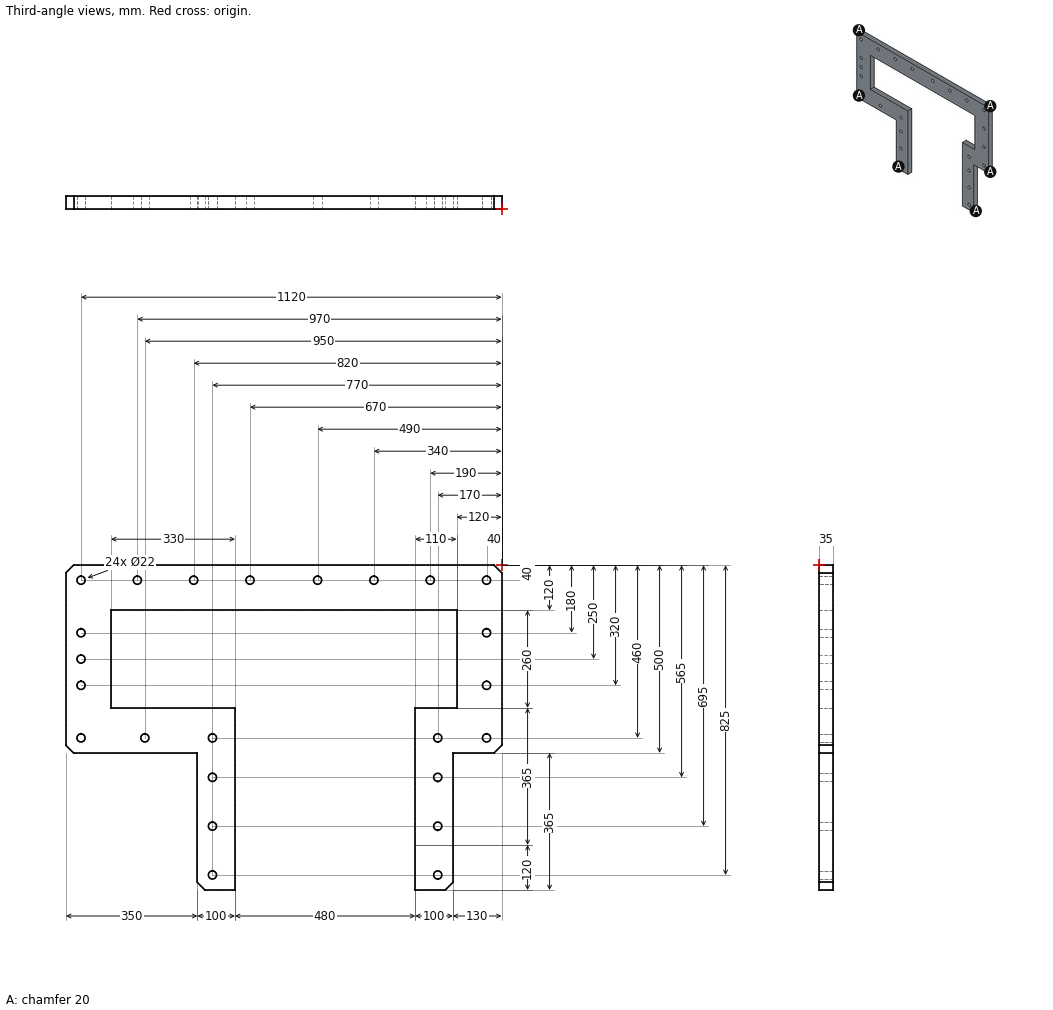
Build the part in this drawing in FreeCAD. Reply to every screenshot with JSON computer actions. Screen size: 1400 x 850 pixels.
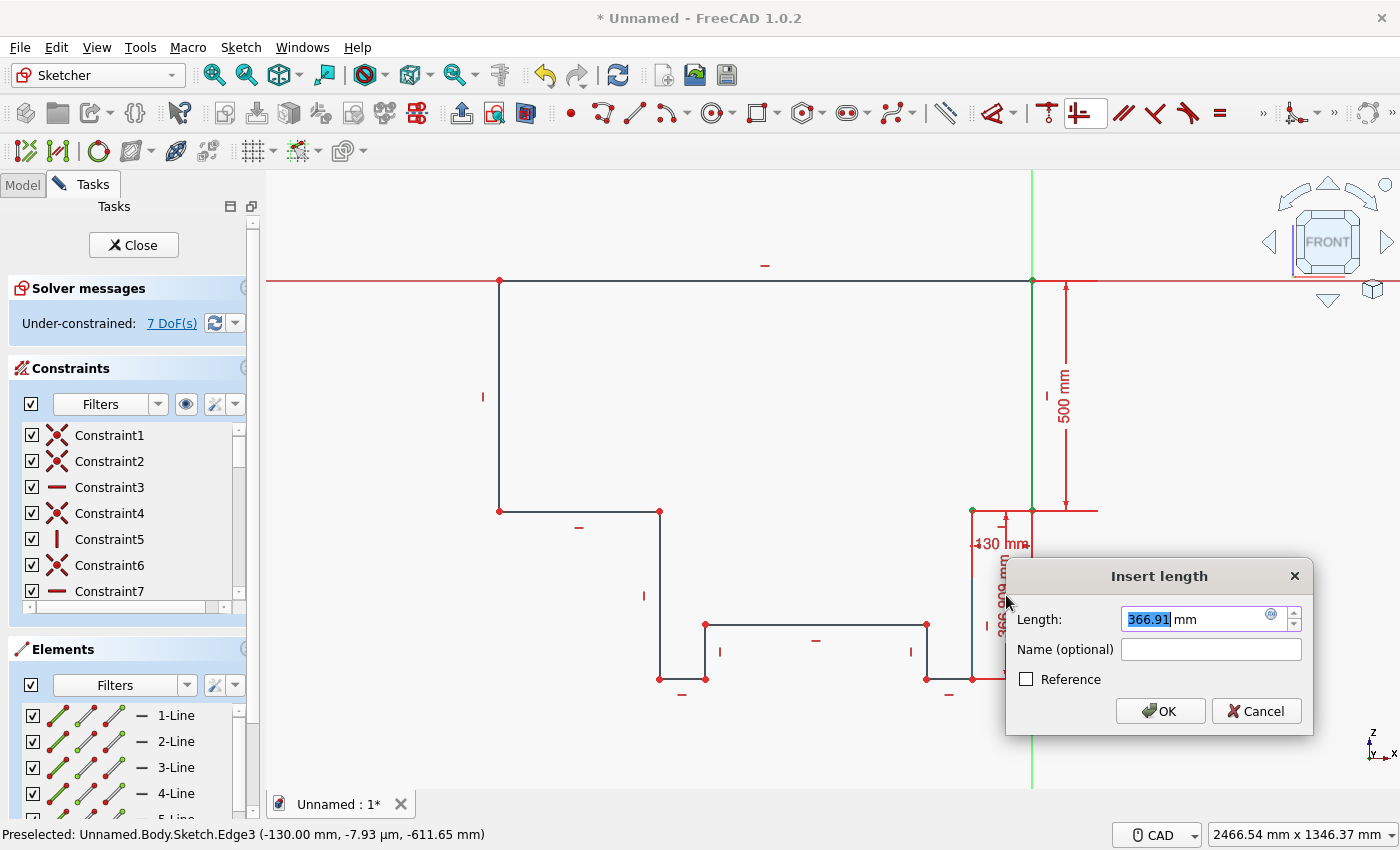
{"action": "type", "text": "365"}
{"action": "key", "text": "Return"}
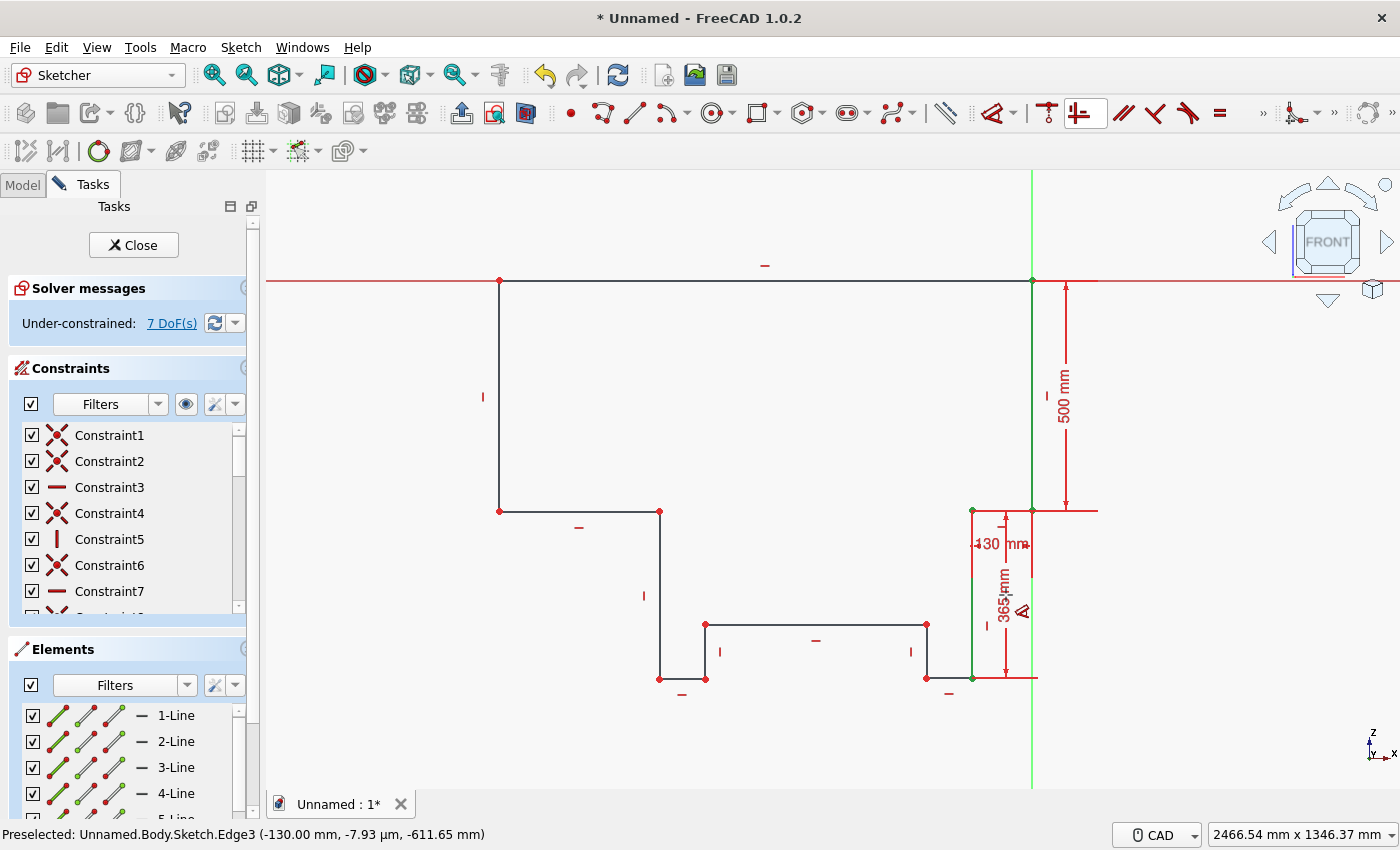
{"action": "left_click", "coordinate": [959, 678]}
{"action": "left_click", "coordinate": [949, 712]}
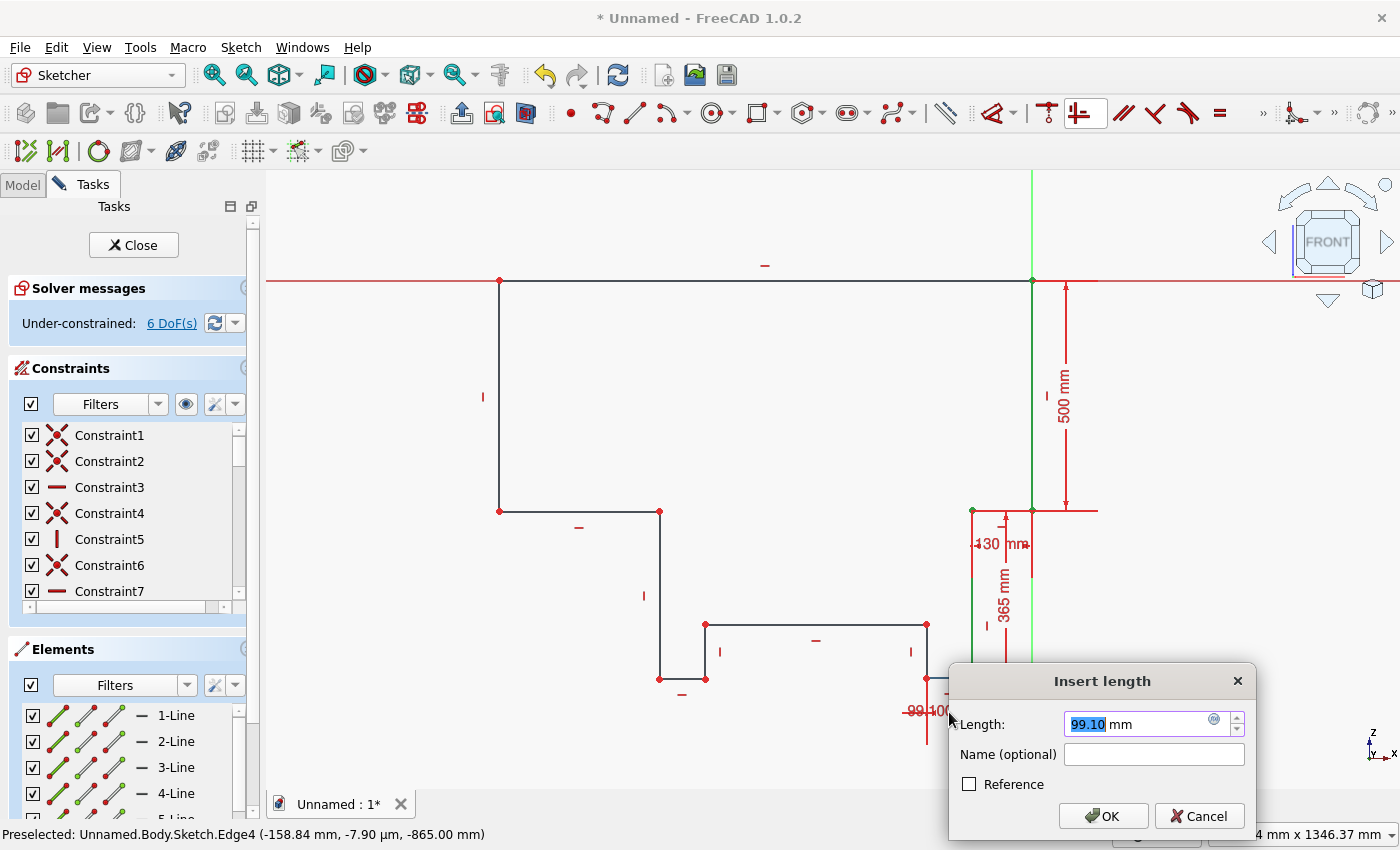
{"action": "type", "text": "100"}
{"action": "key", "text": "Return"}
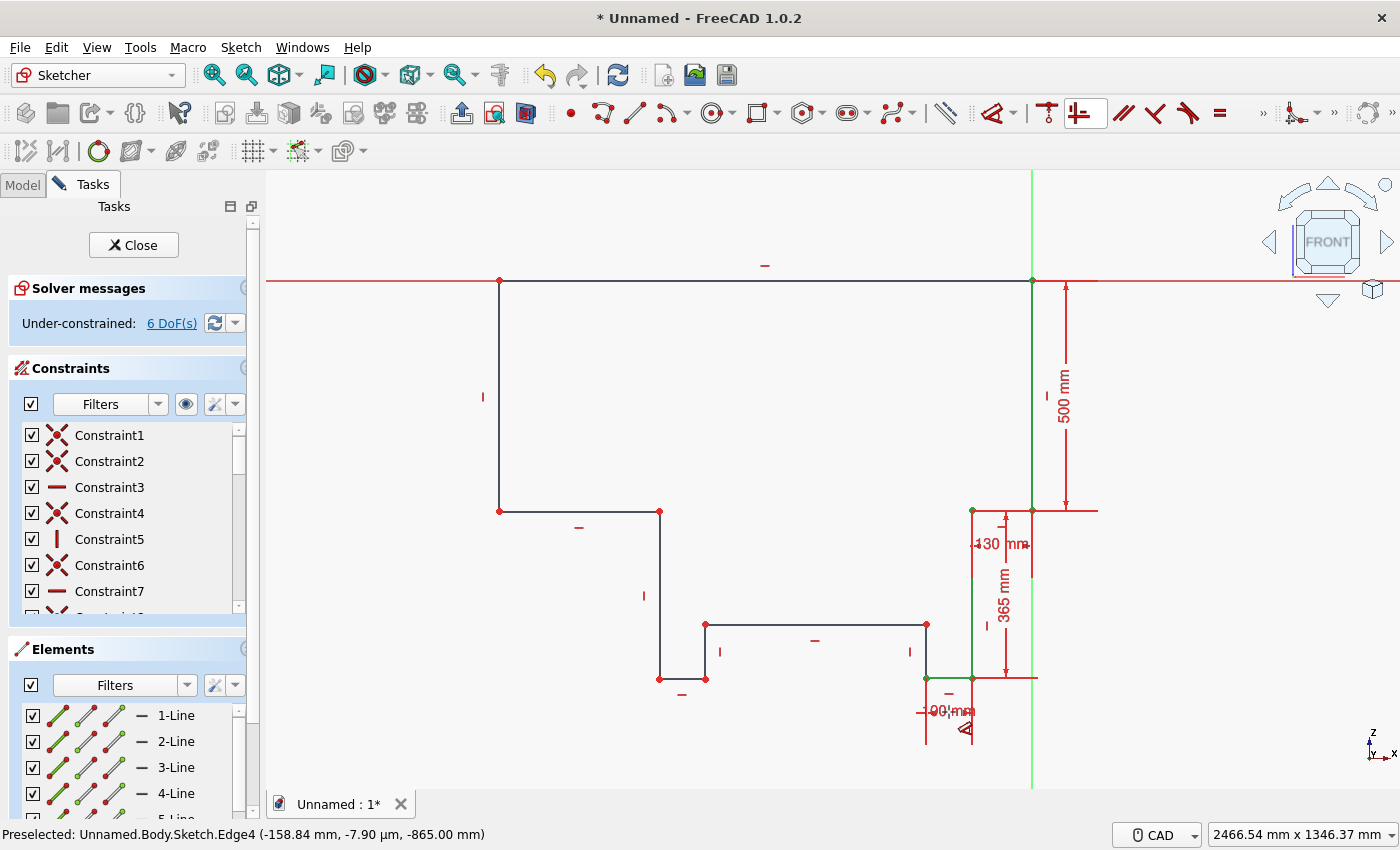
{"action": "left_click", "coordinate": [926, 662]}
{"action": "left_click", "coordinate": [892, 652]}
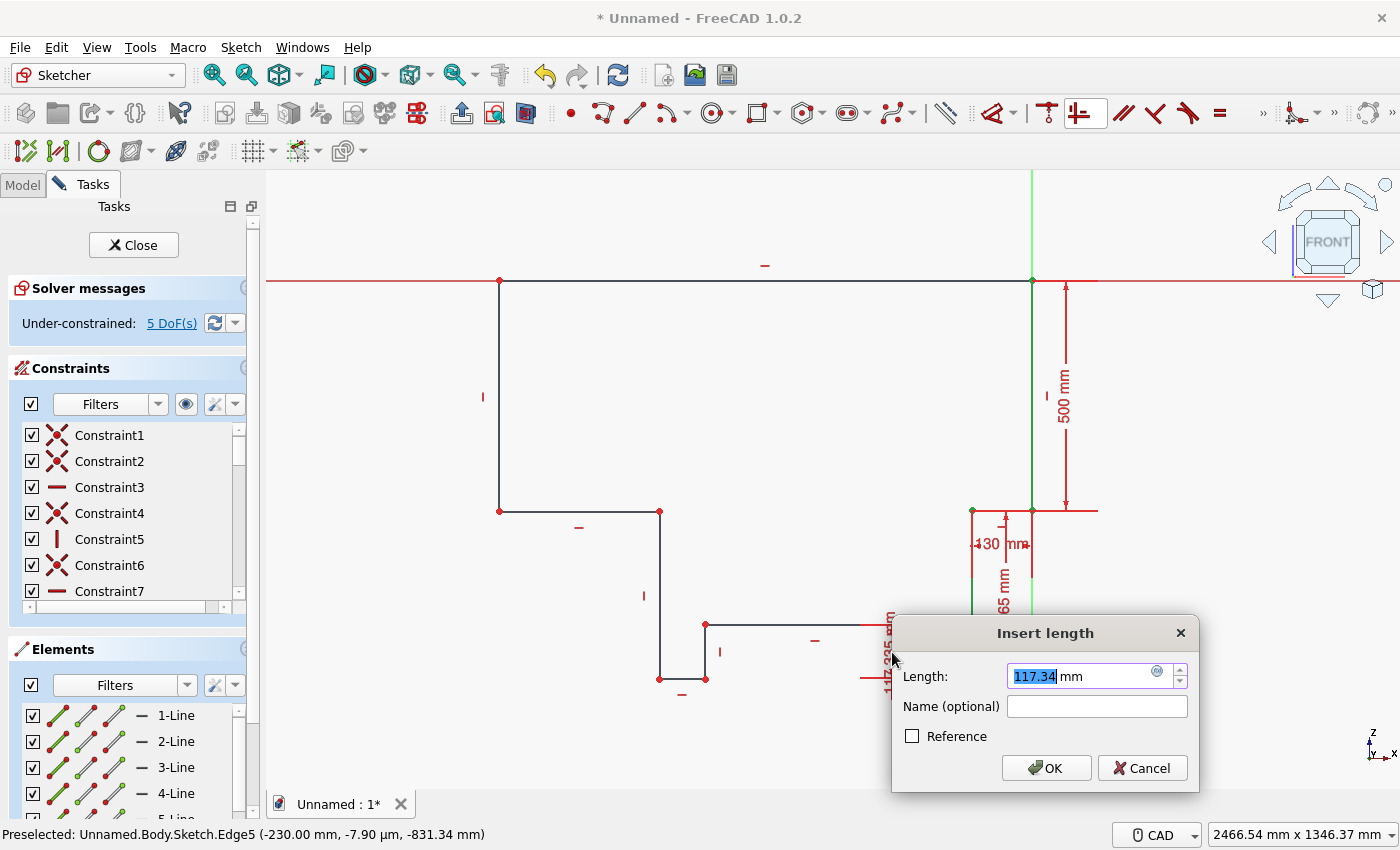
{"action": "type", "text": "120"}
{"action": "key", "text": "Return"}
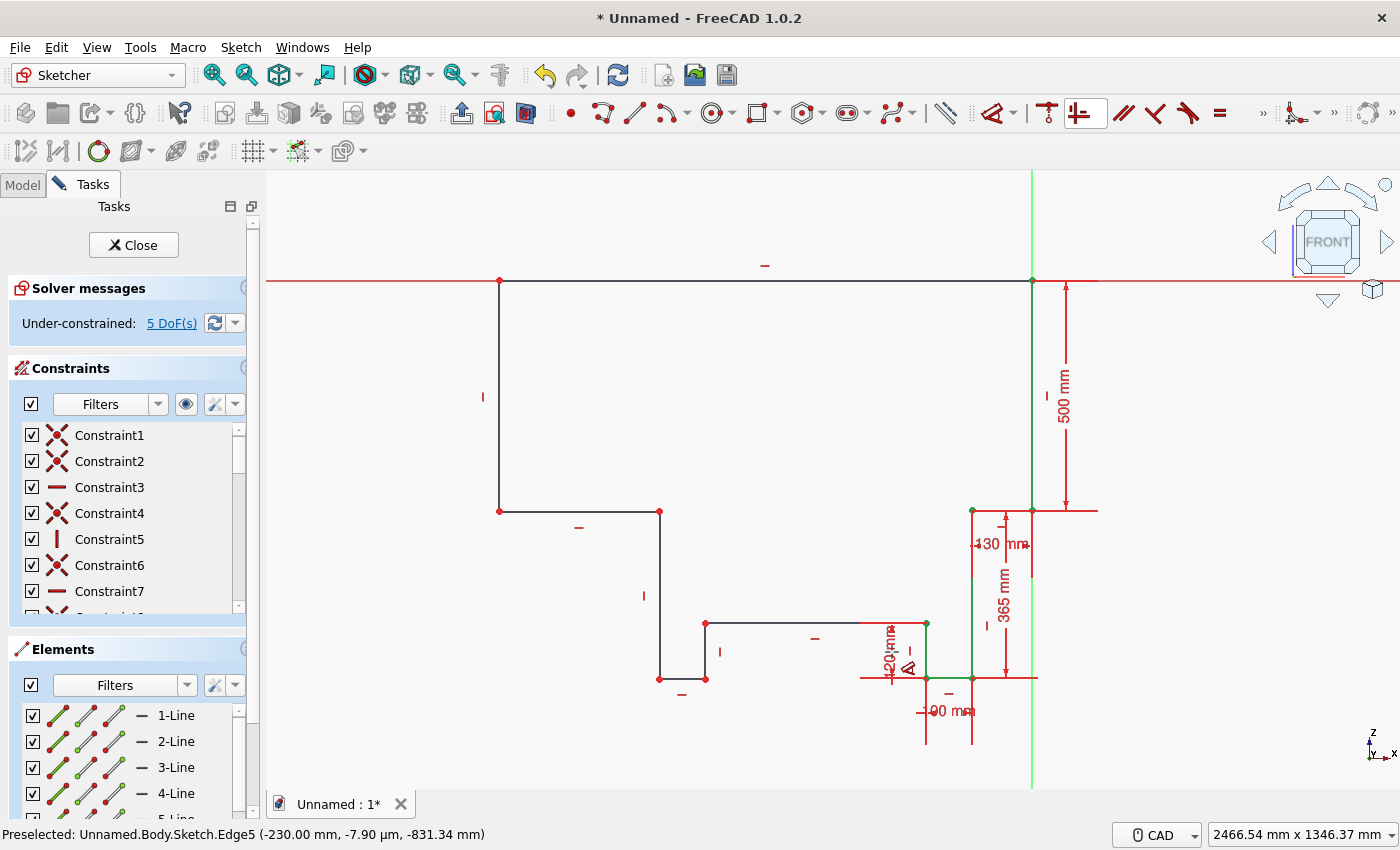
{"action": "left_click", "coordinate": [860, 623]}
{"action": "left_click", "coordinate": [816, 657]}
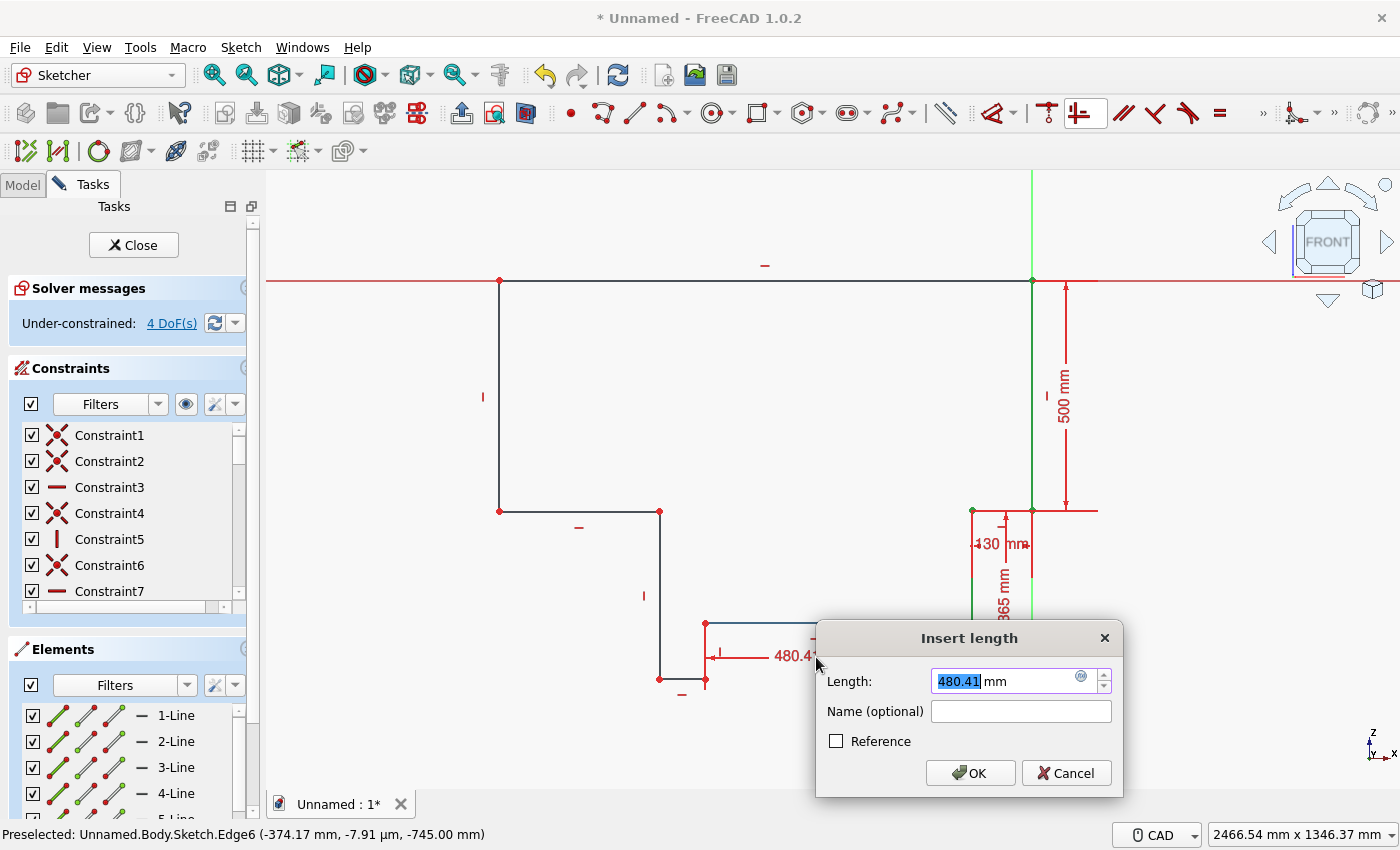
{"action": "type", "text": "480"}
{"action": "key", "text": "Return"}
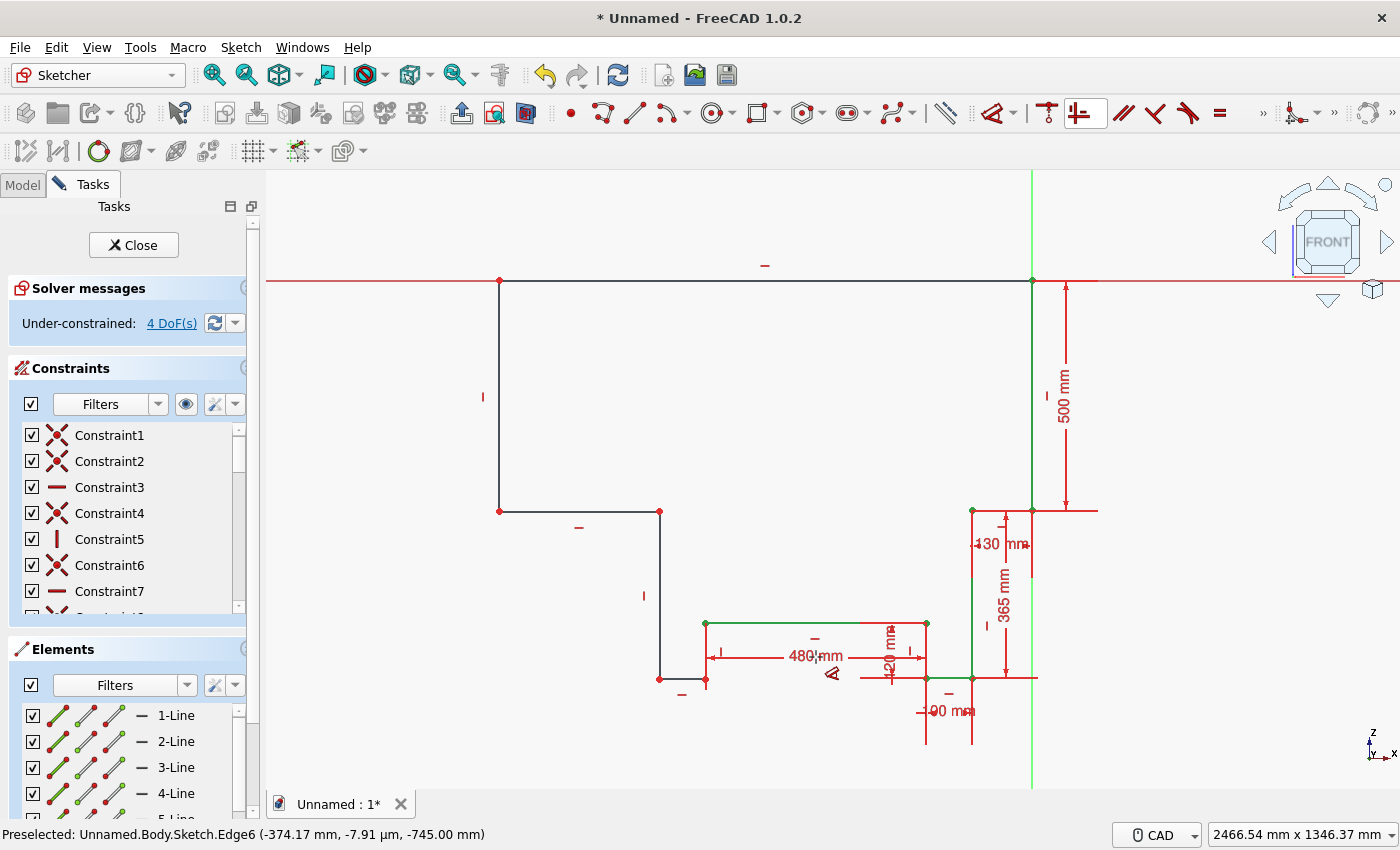
{"action": "left_click", "coordinate": [706, 640]}
{"action": "left_click", "coordinate": [740, 651]}